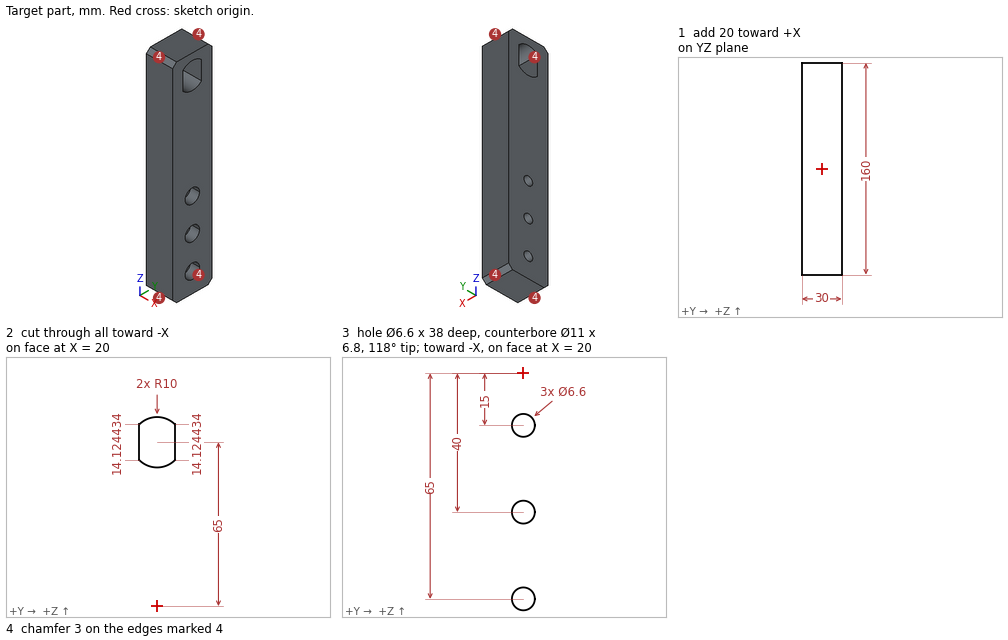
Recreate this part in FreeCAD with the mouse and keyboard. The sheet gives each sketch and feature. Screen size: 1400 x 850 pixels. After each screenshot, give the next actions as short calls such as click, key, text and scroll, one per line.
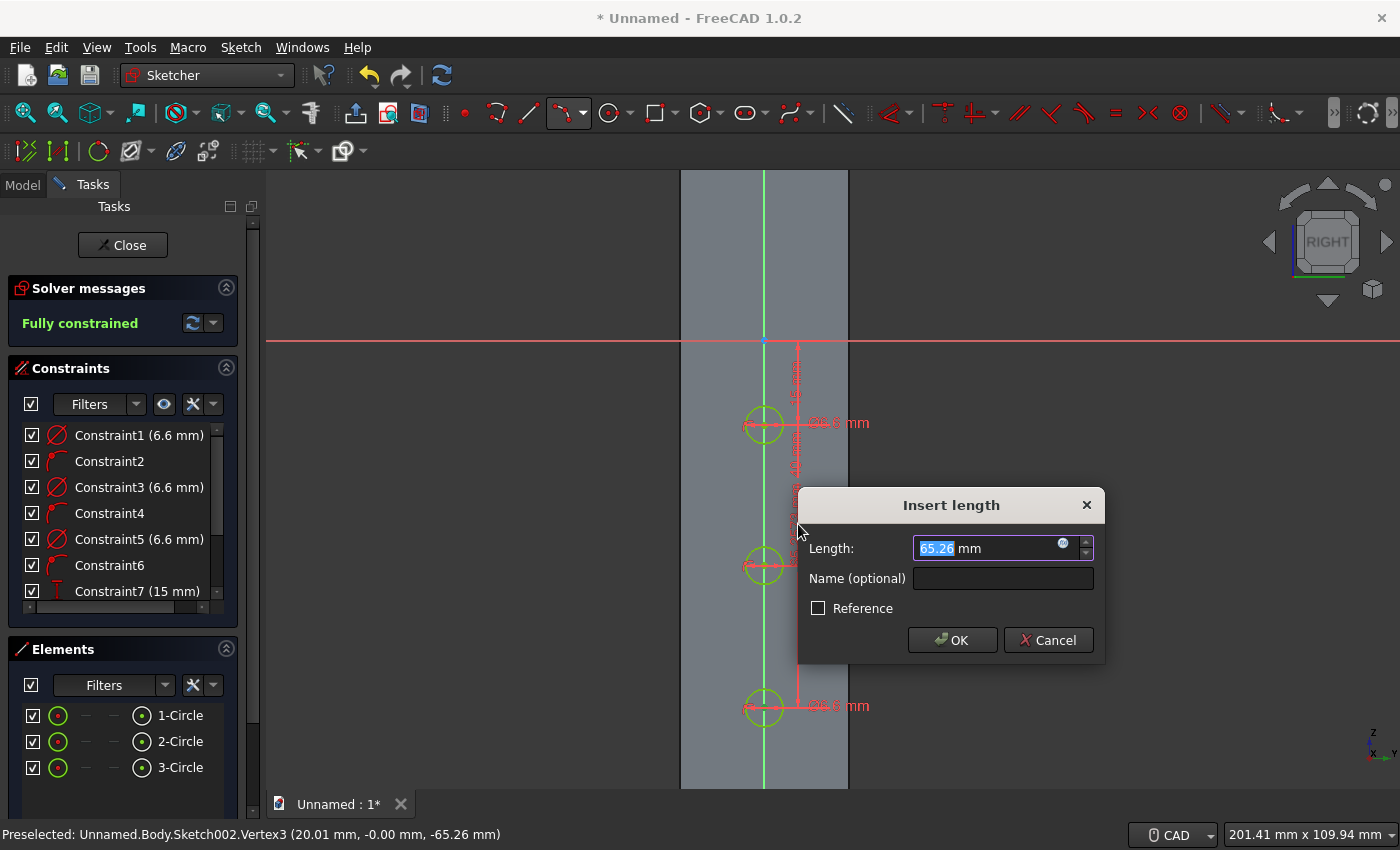
text(65)
key(Return)
key(Escape)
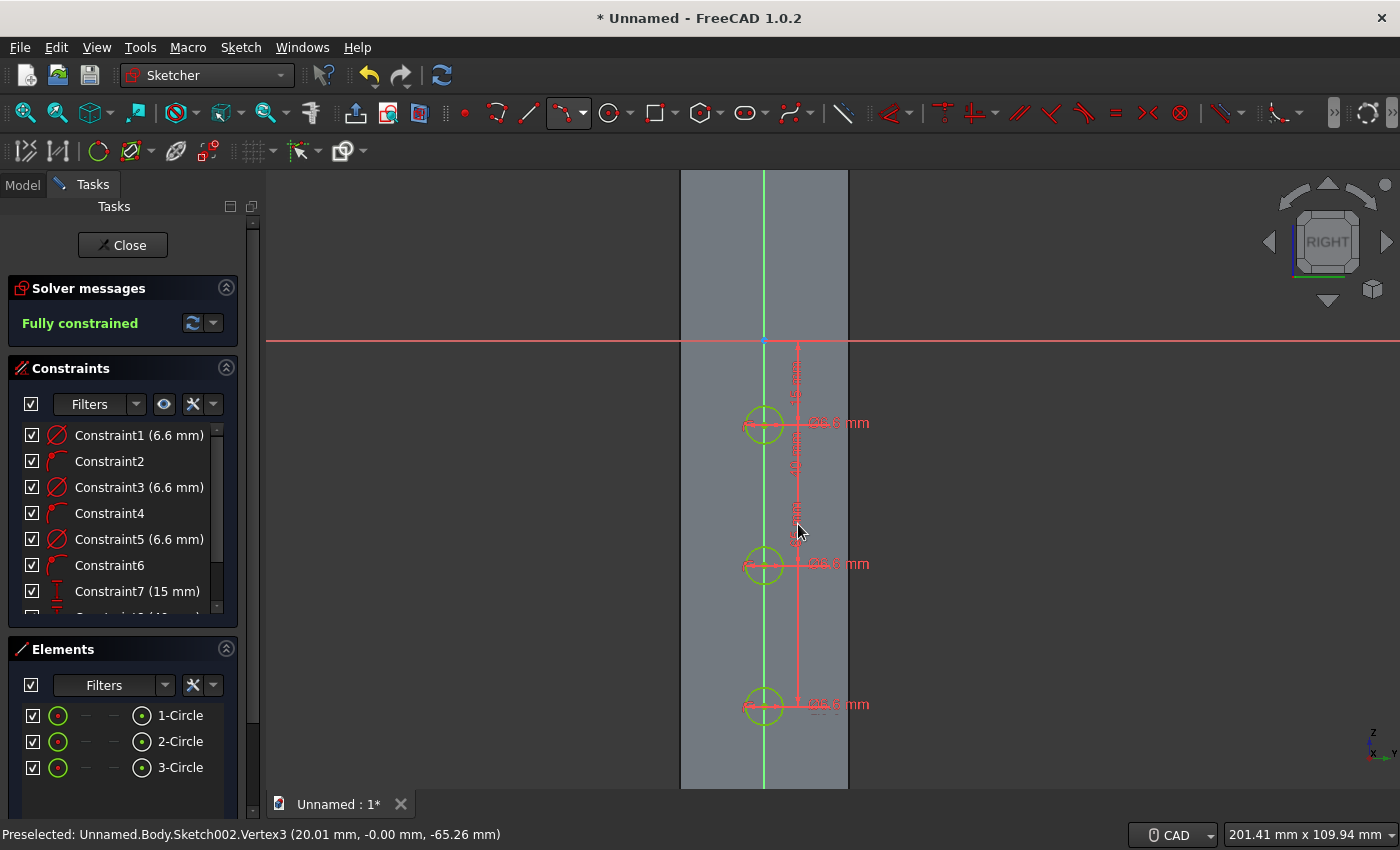
click(123, 245)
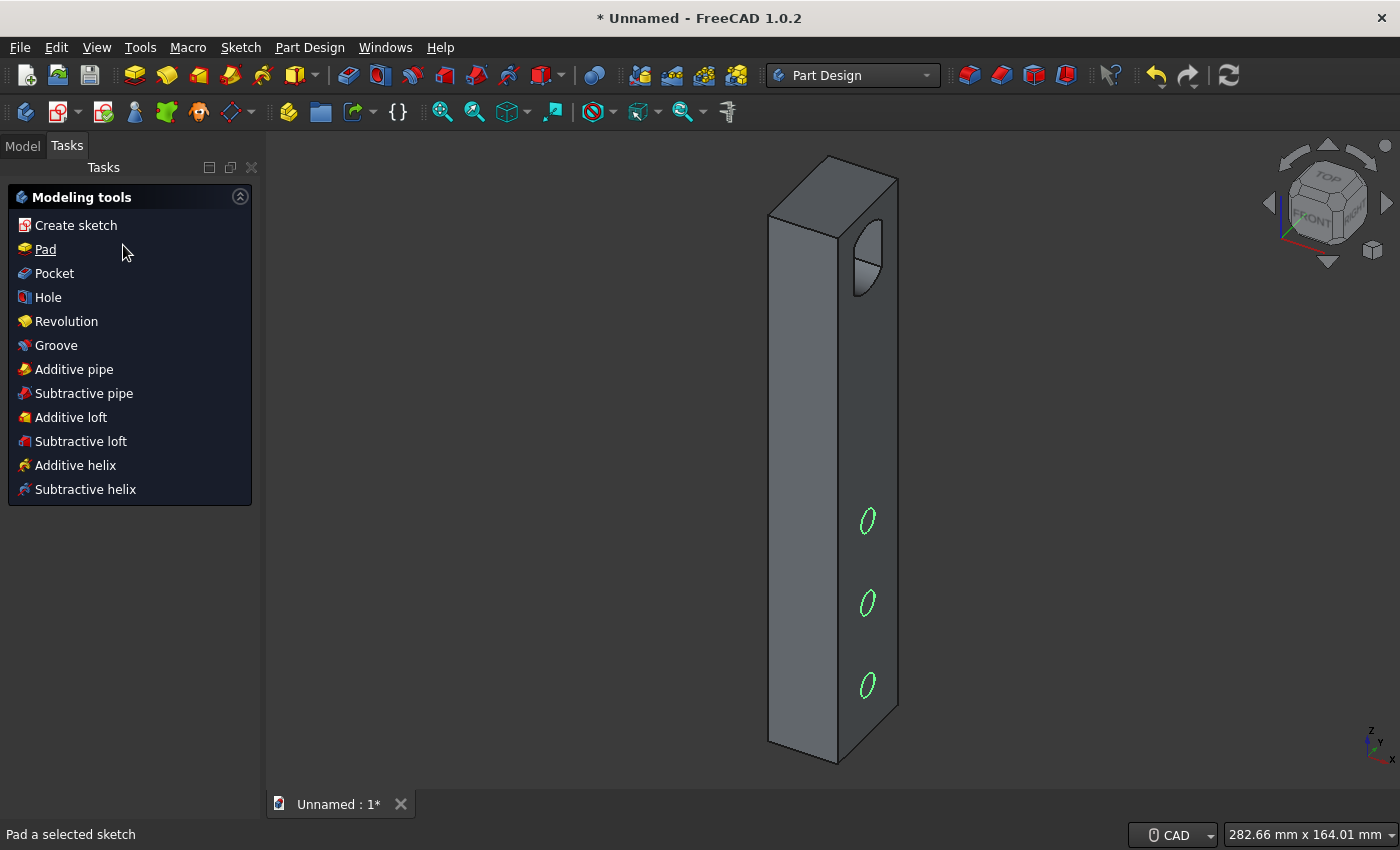
click(382, 76)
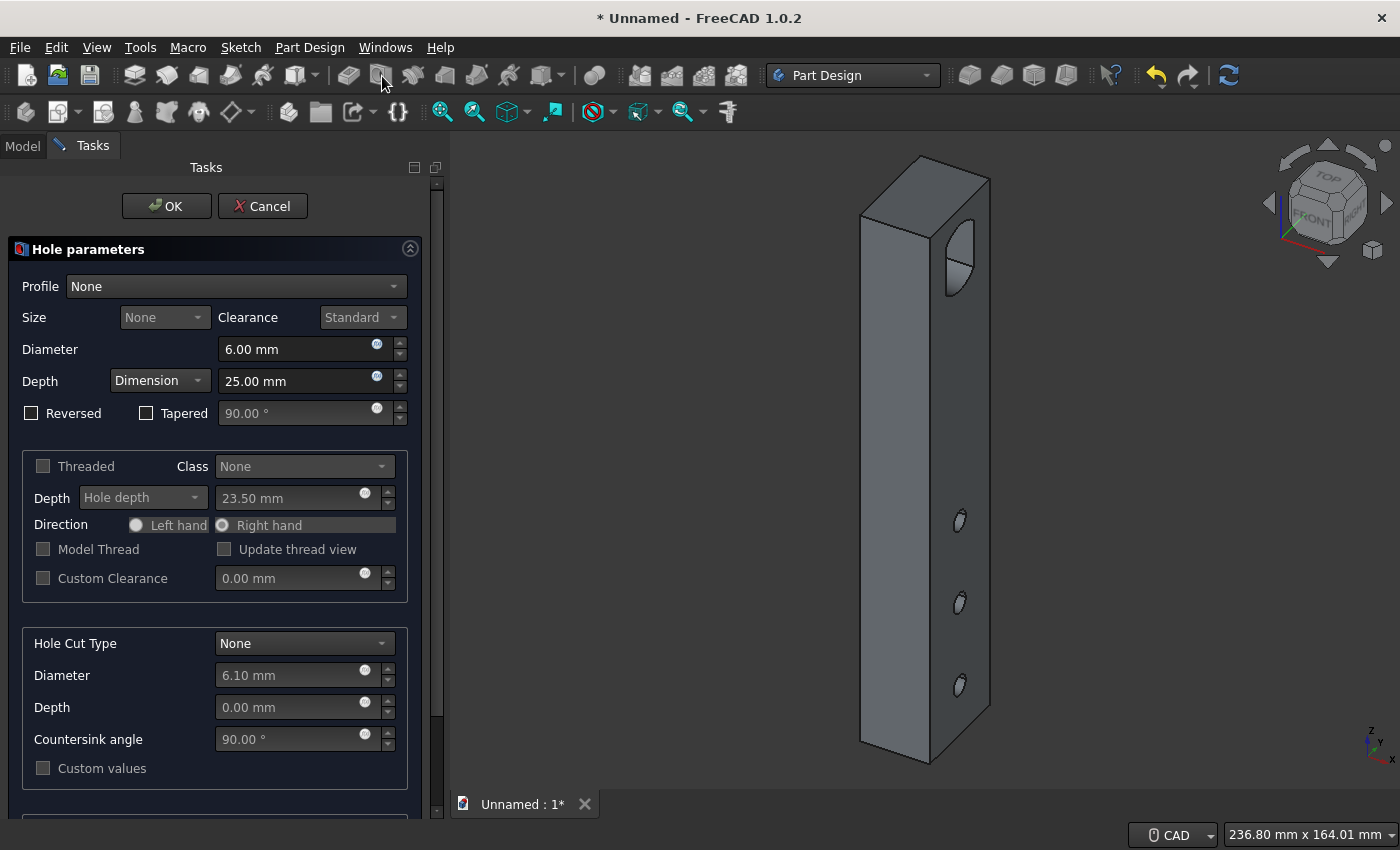
triple_click(305, 349)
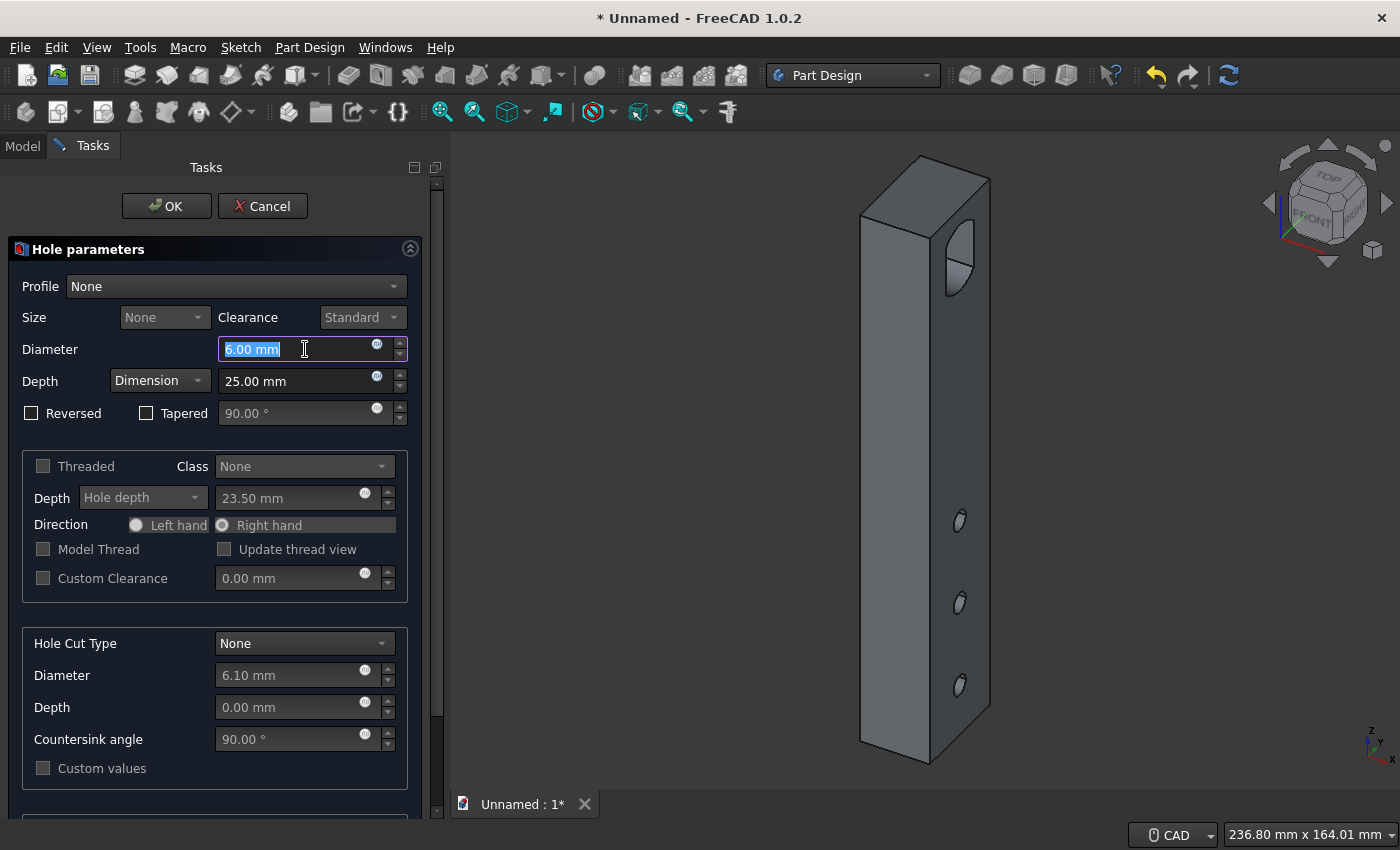
text(6.6)
key(Tab)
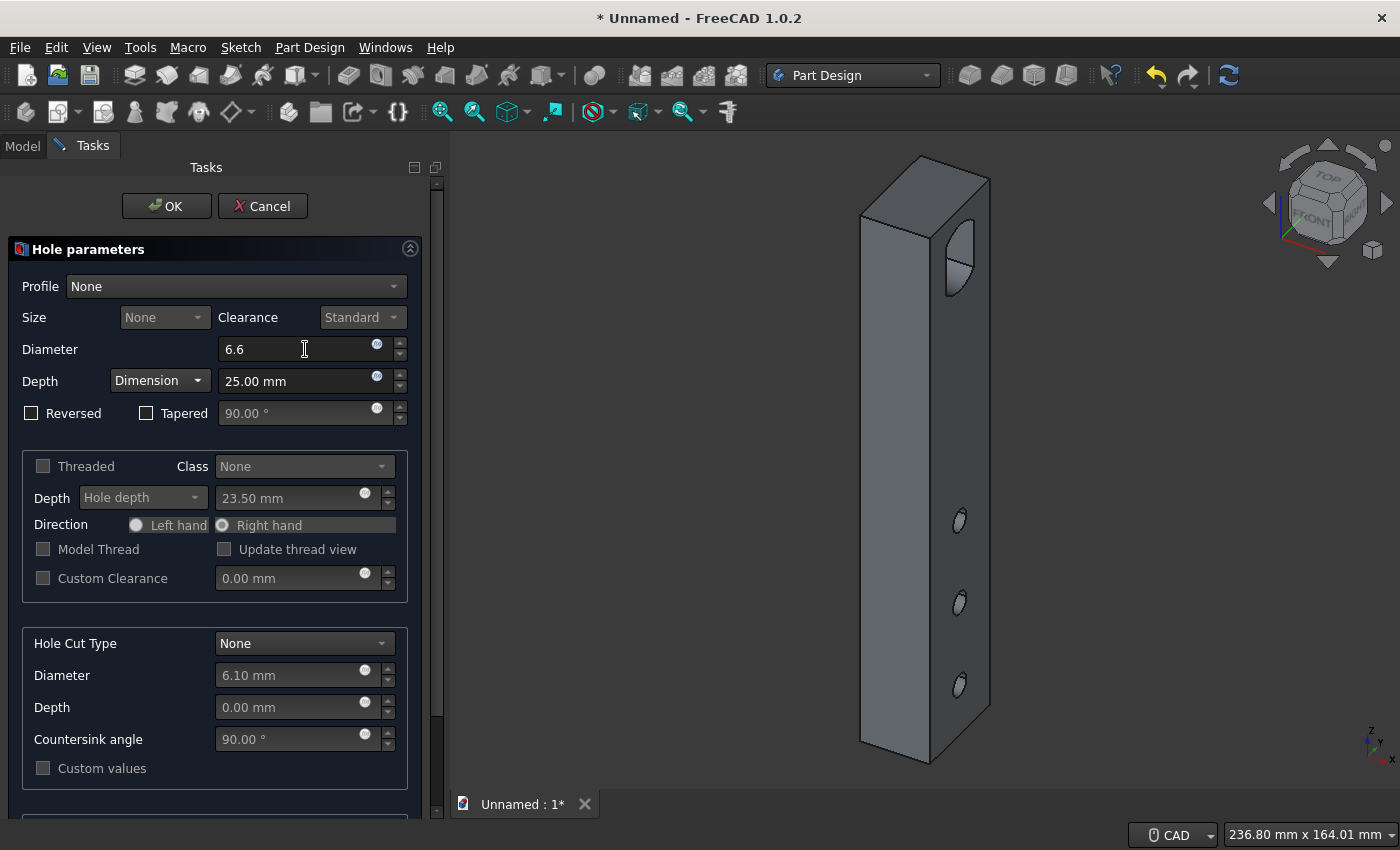
triple_click(305, 381)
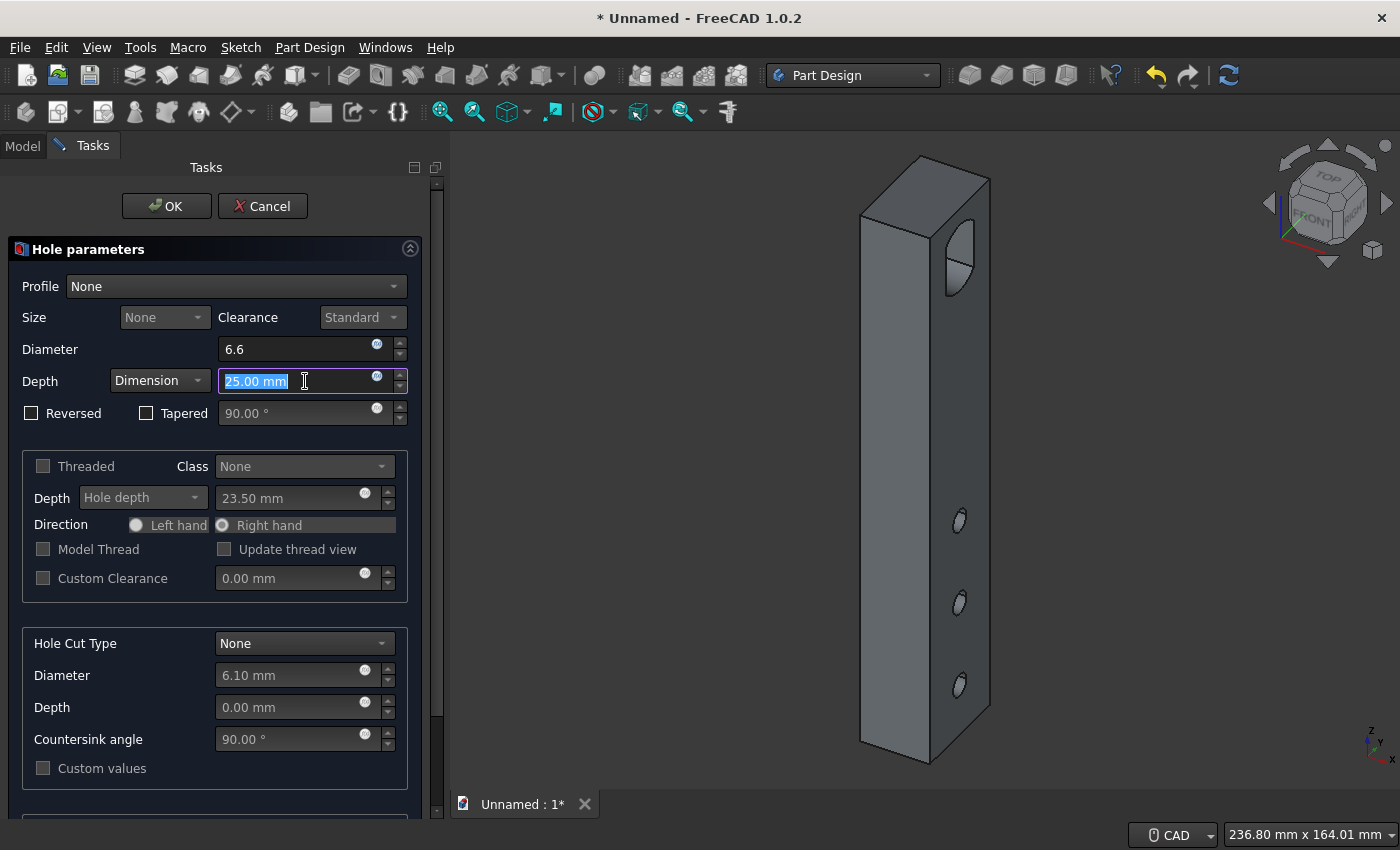
text(38)
key(Tab)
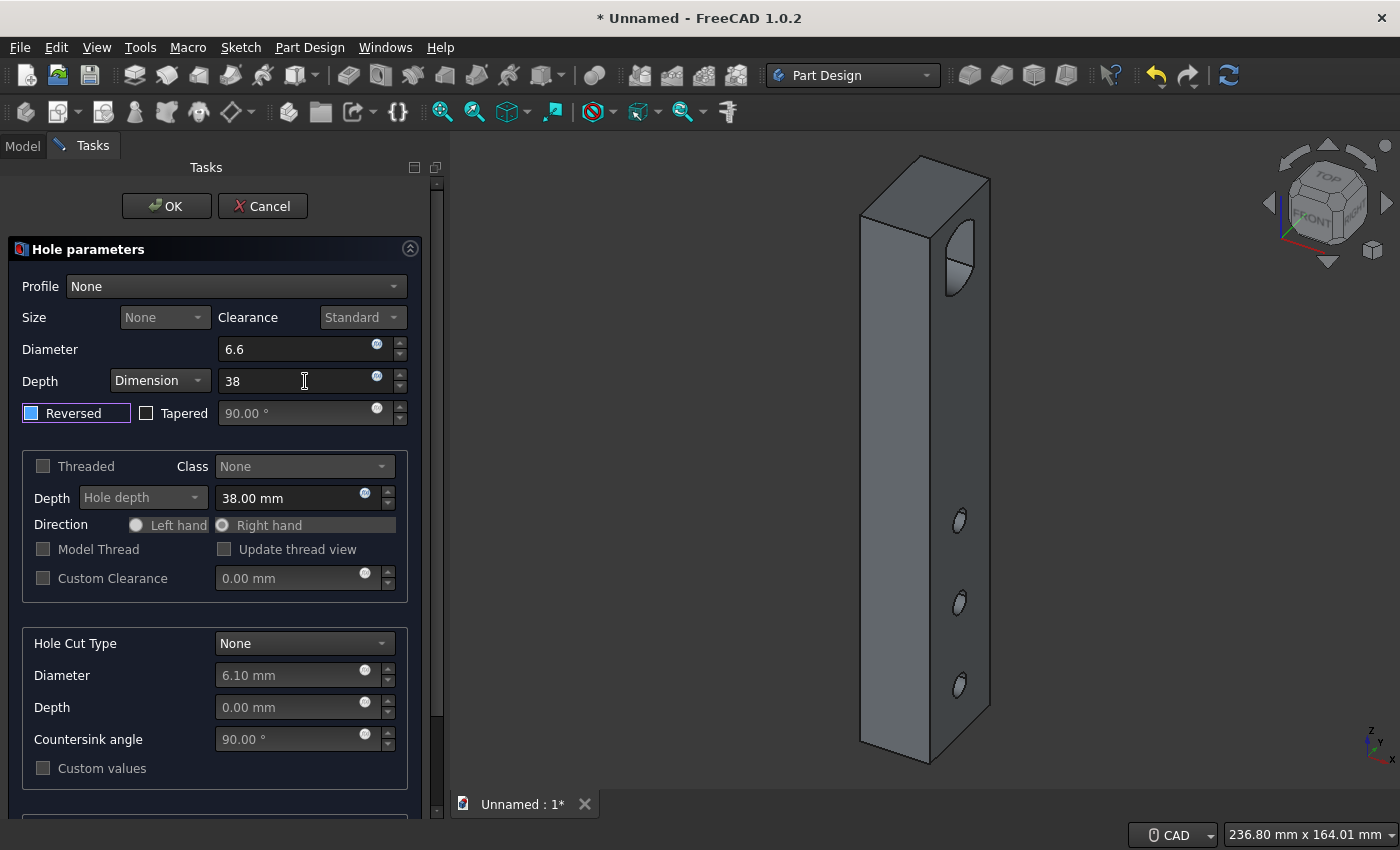
click(306, 644)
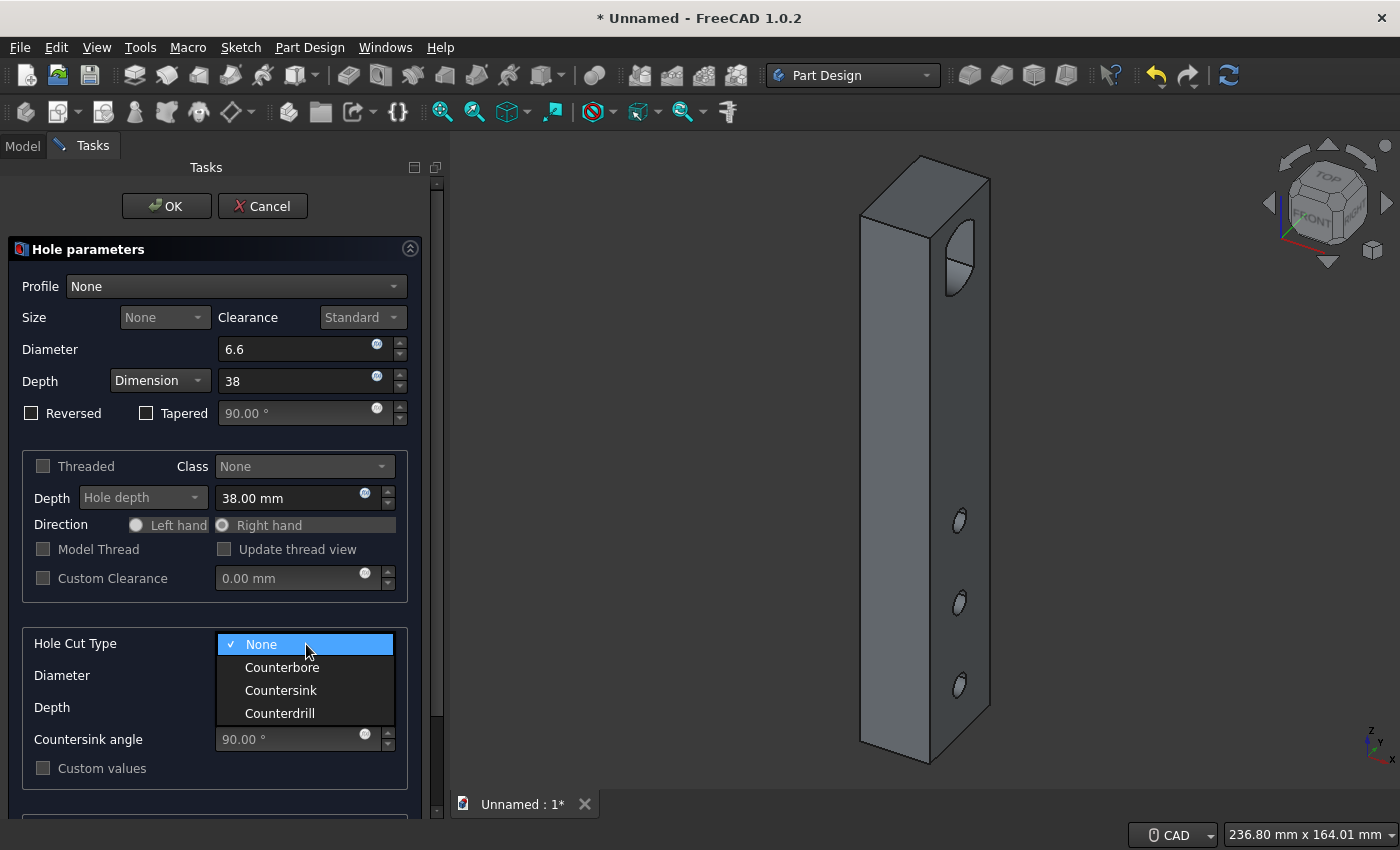
click(304, 668)